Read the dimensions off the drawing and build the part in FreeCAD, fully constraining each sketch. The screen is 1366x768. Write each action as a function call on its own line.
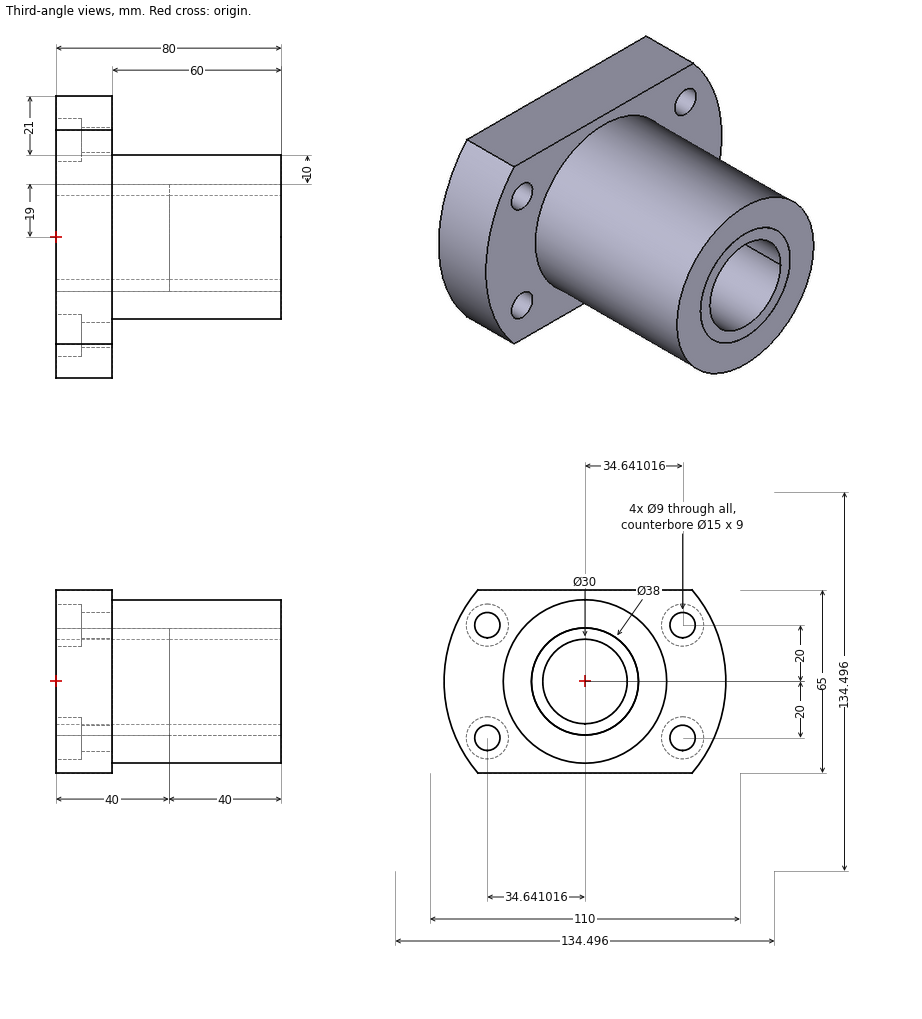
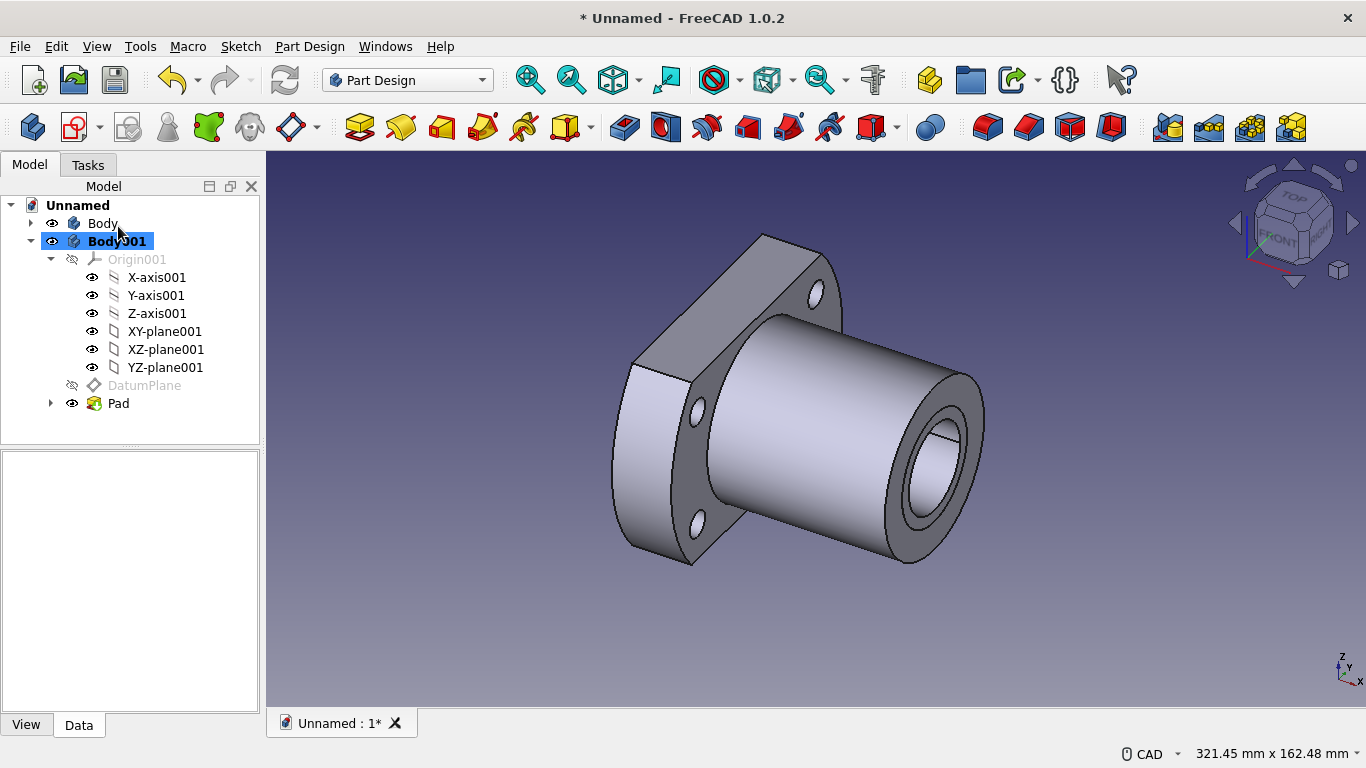
click(531, 80)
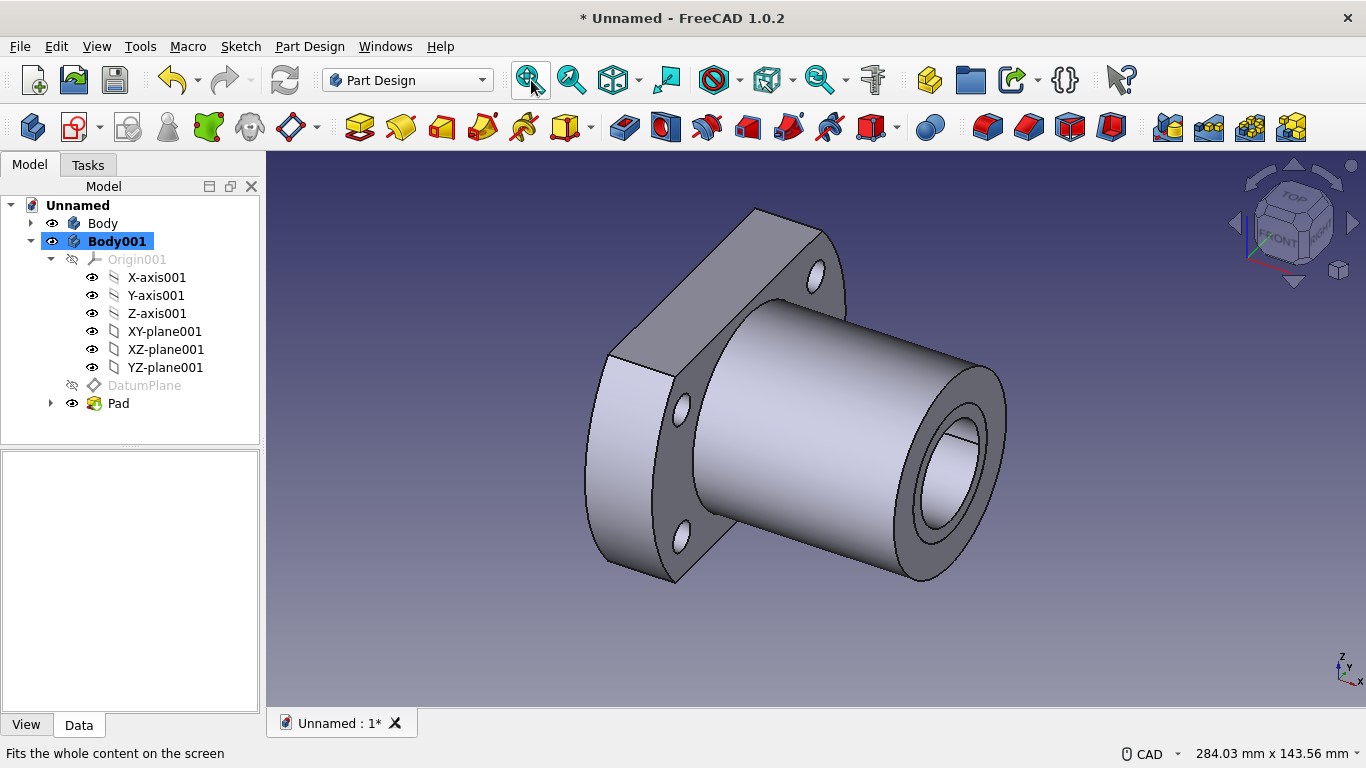
click(33, 128)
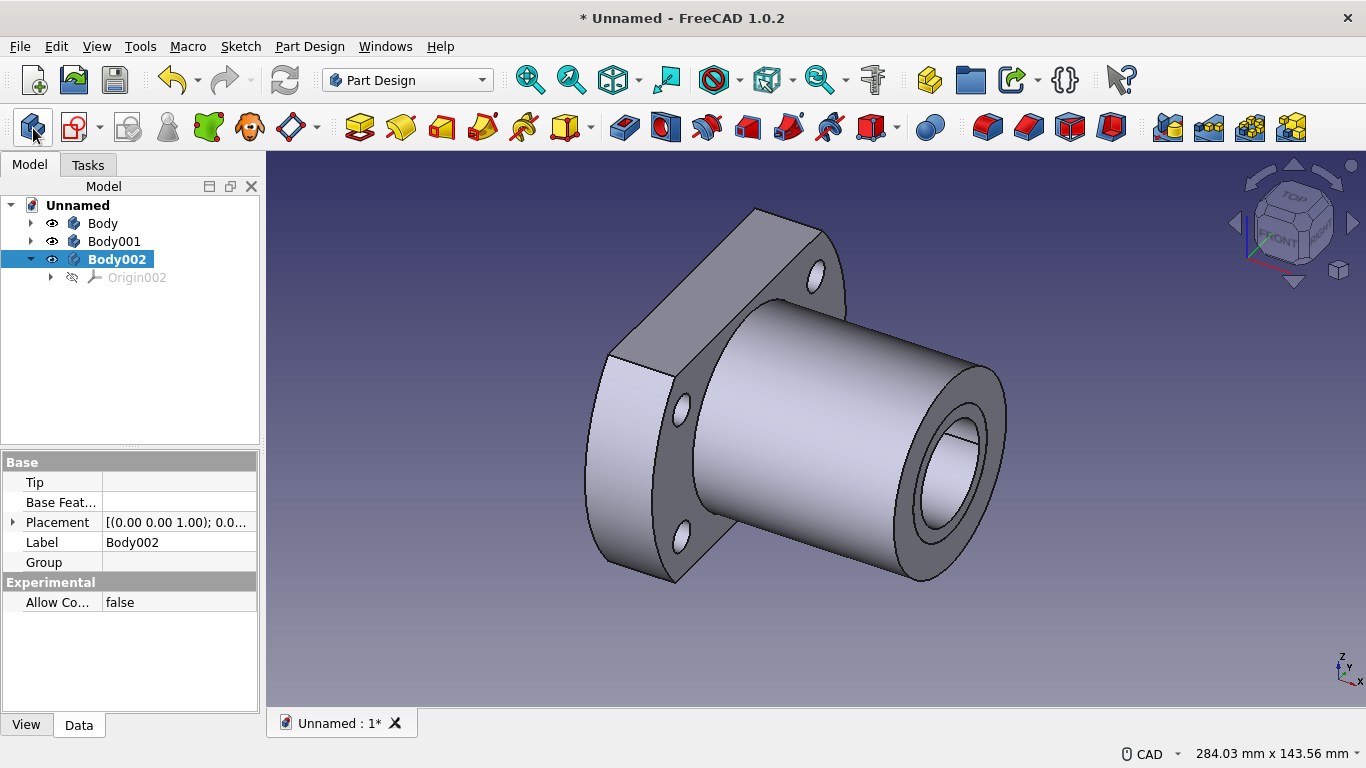
click(306, 667)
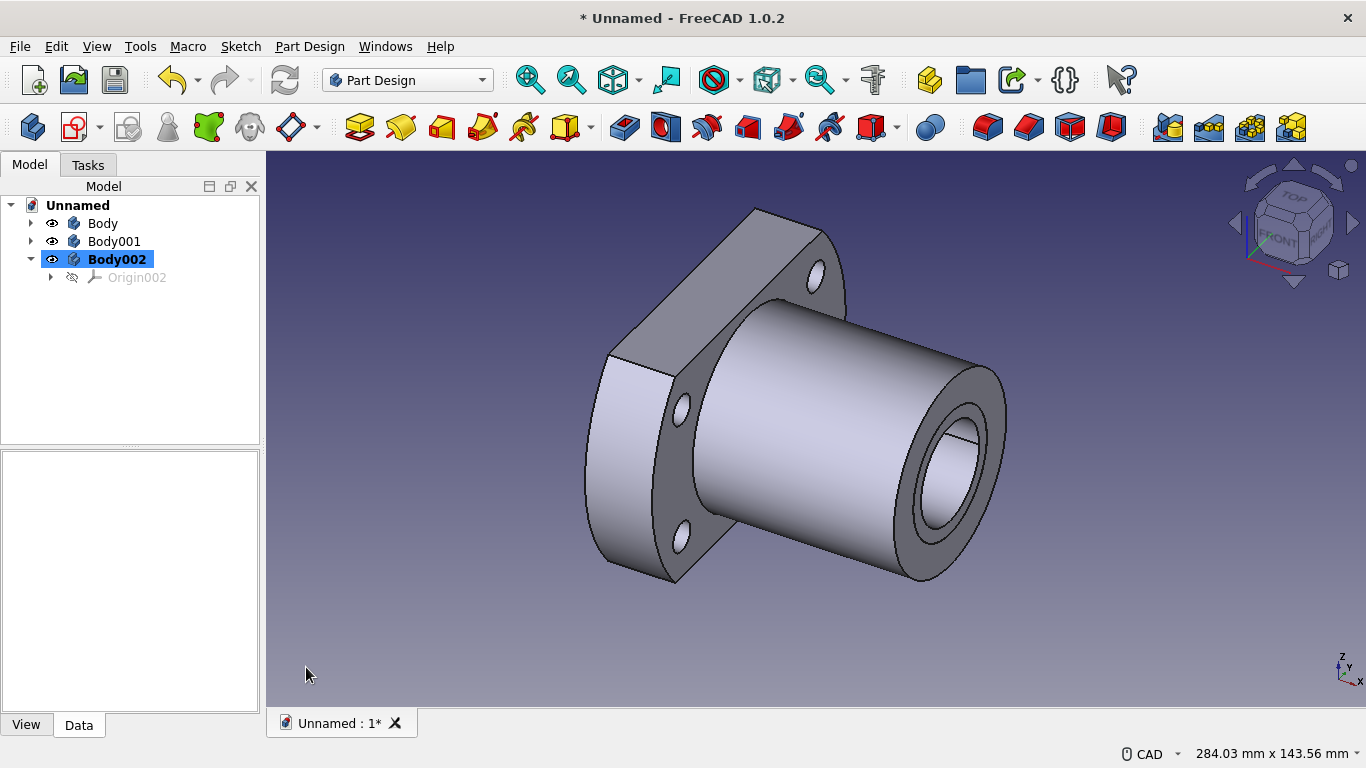
click(74, 128)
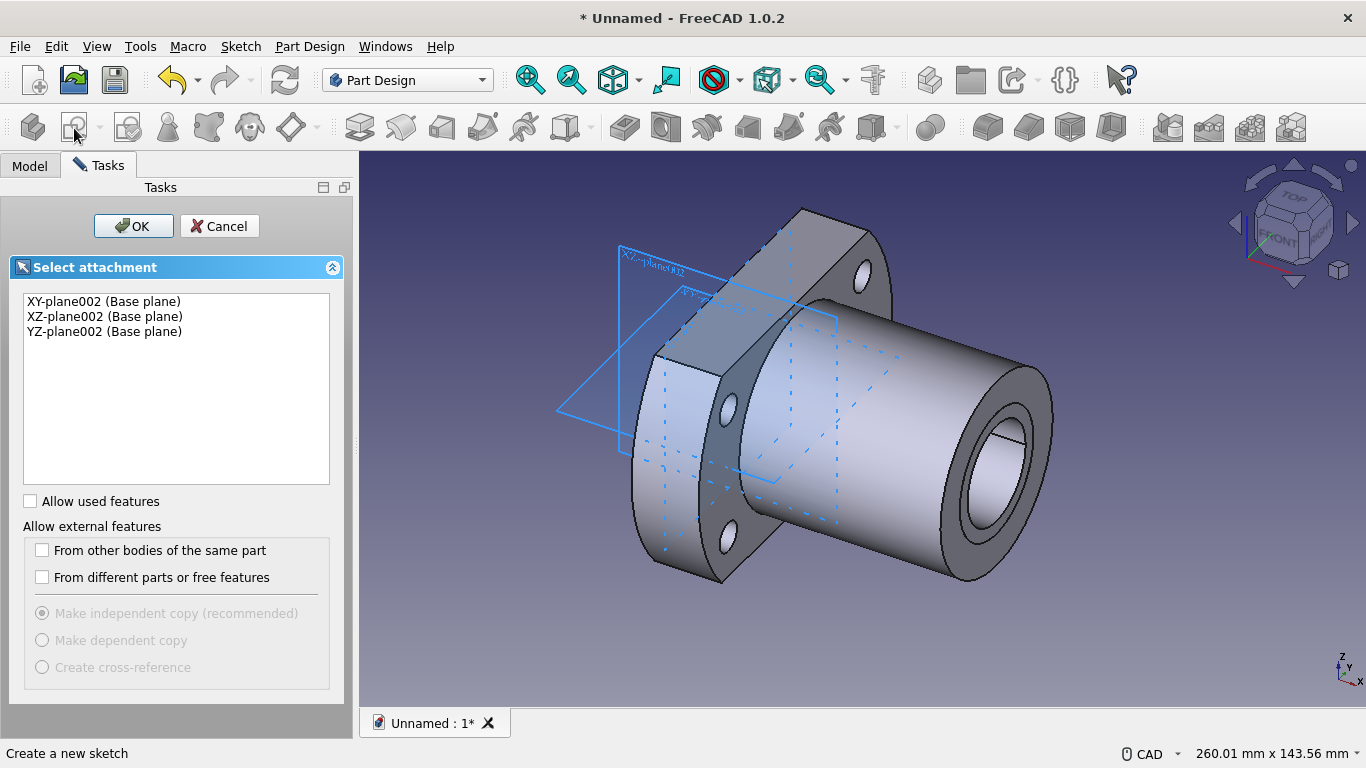
click(84, 332)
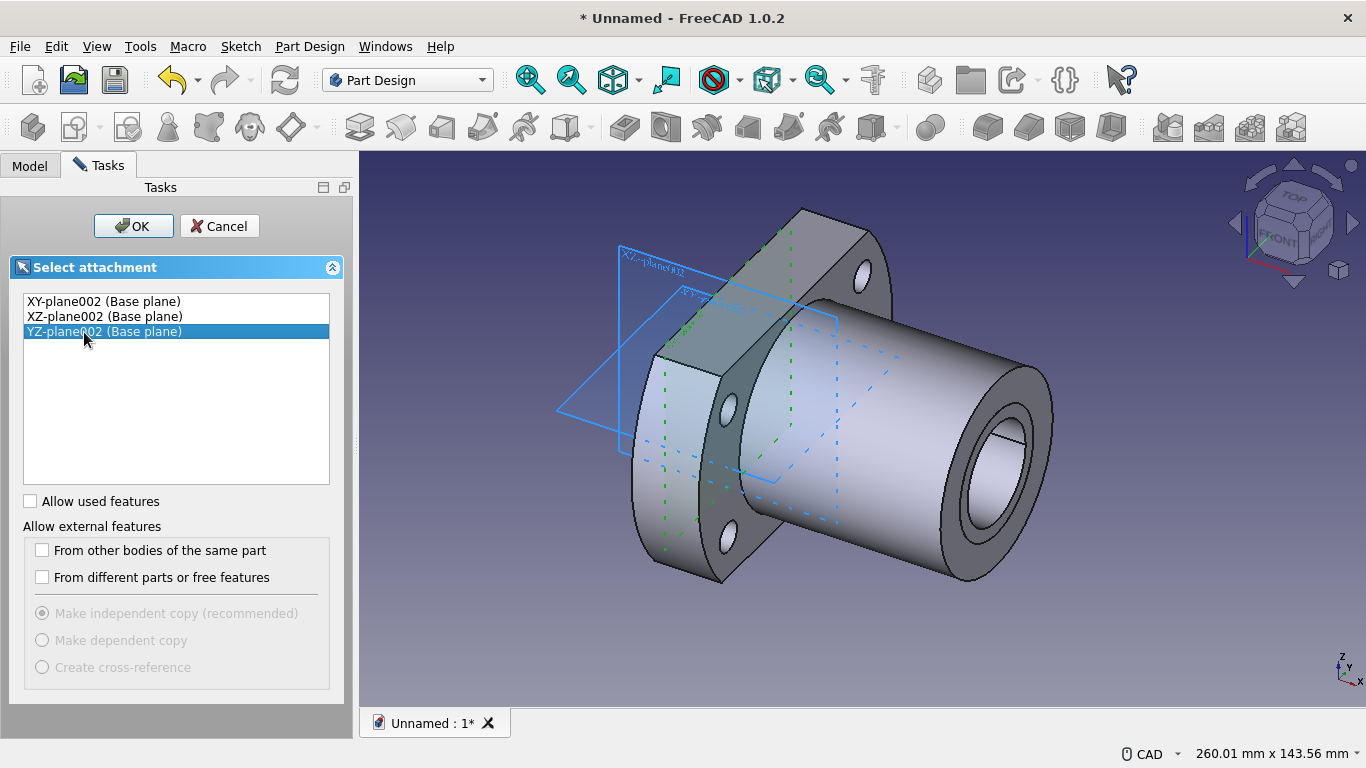
click(134, 226)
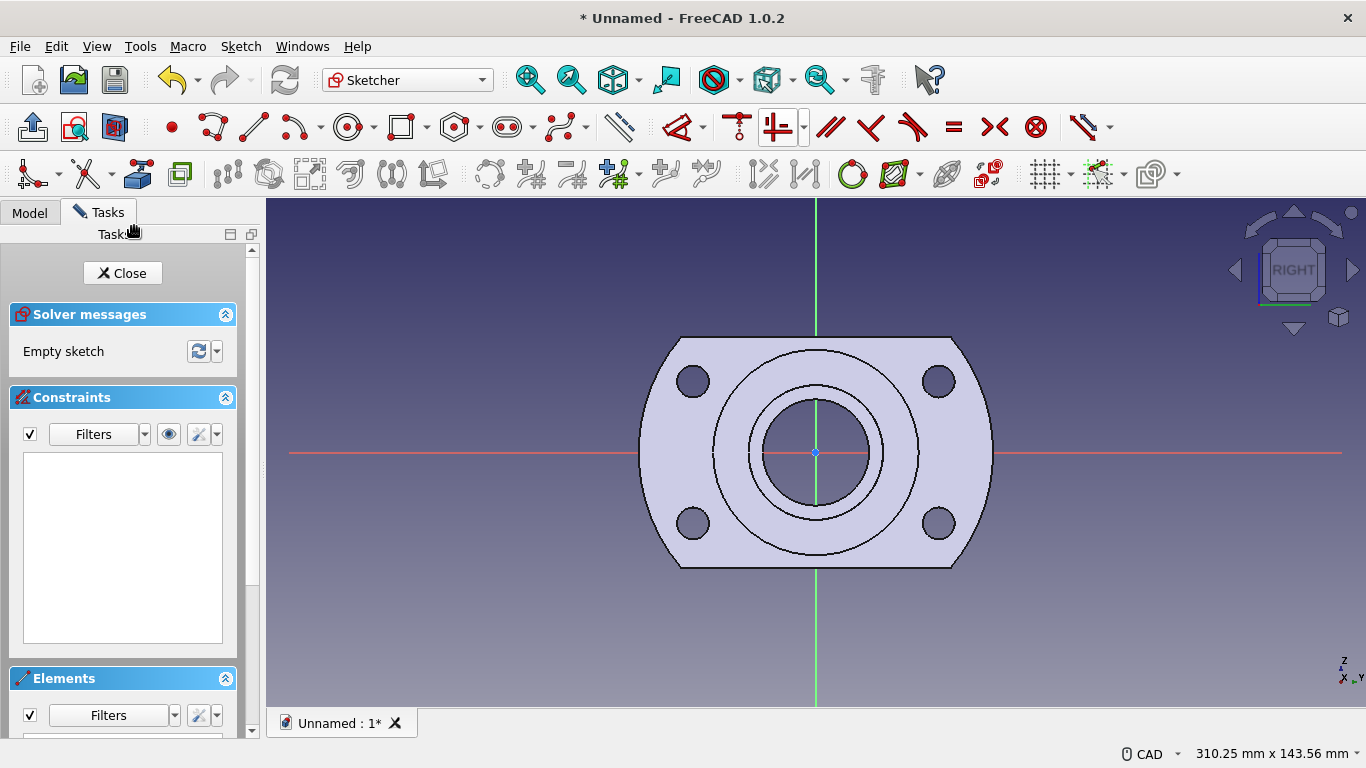
scroll(872, 452, up, 4)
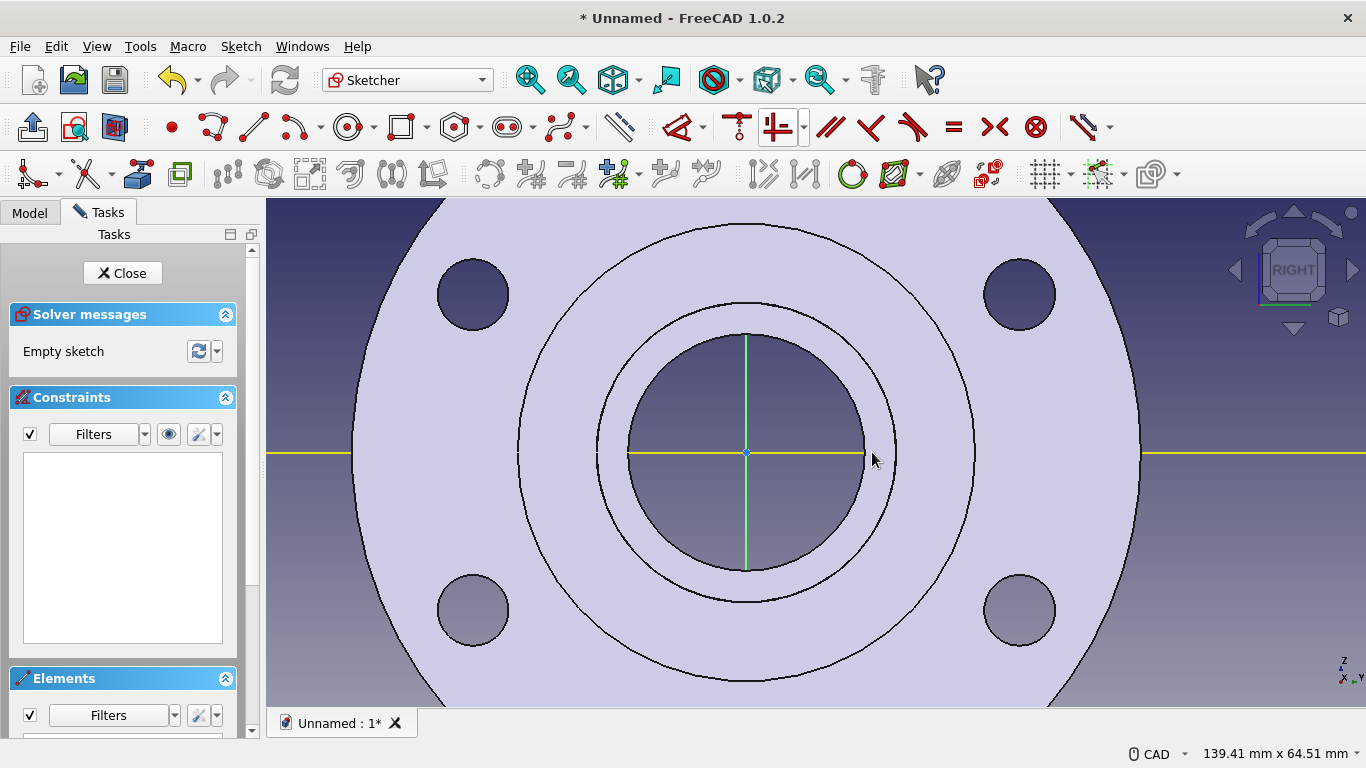
key(g)
key(c)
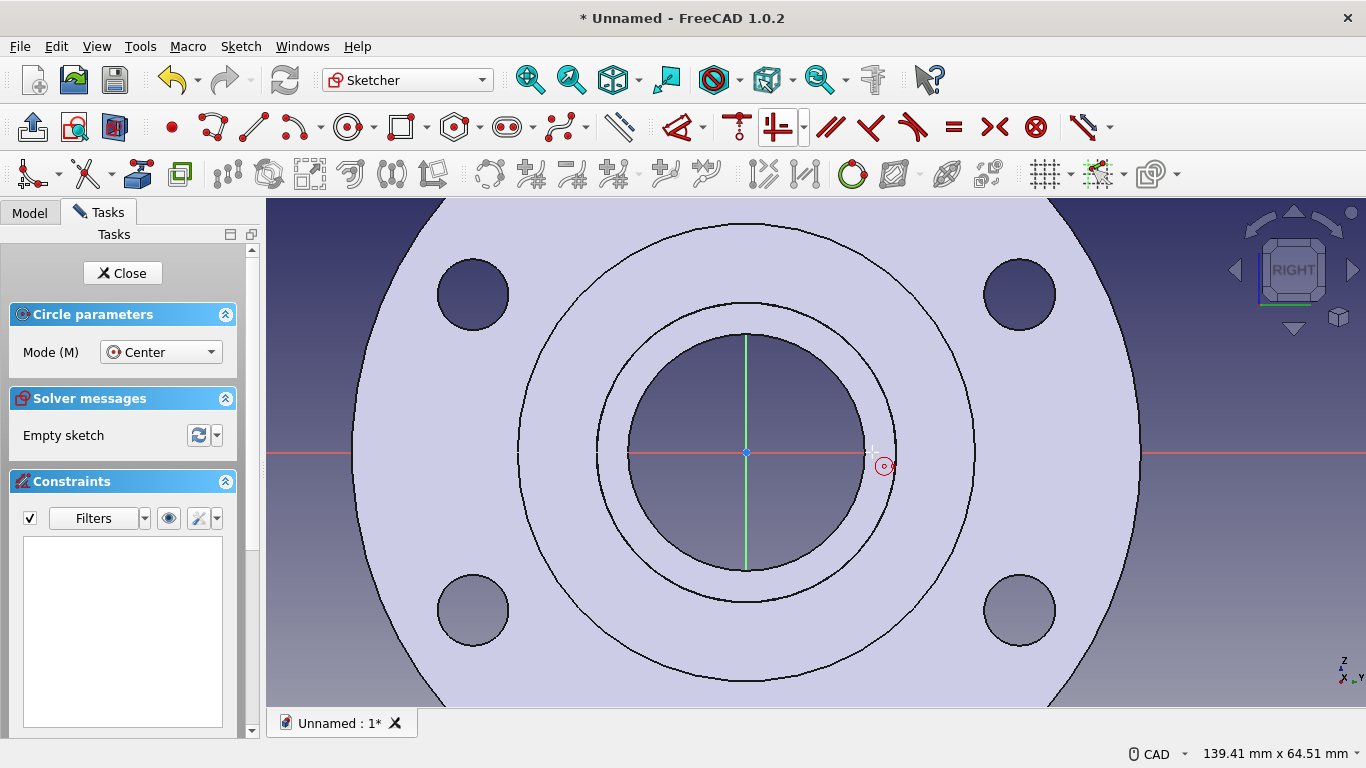
click(746, 452)
click(852, 346)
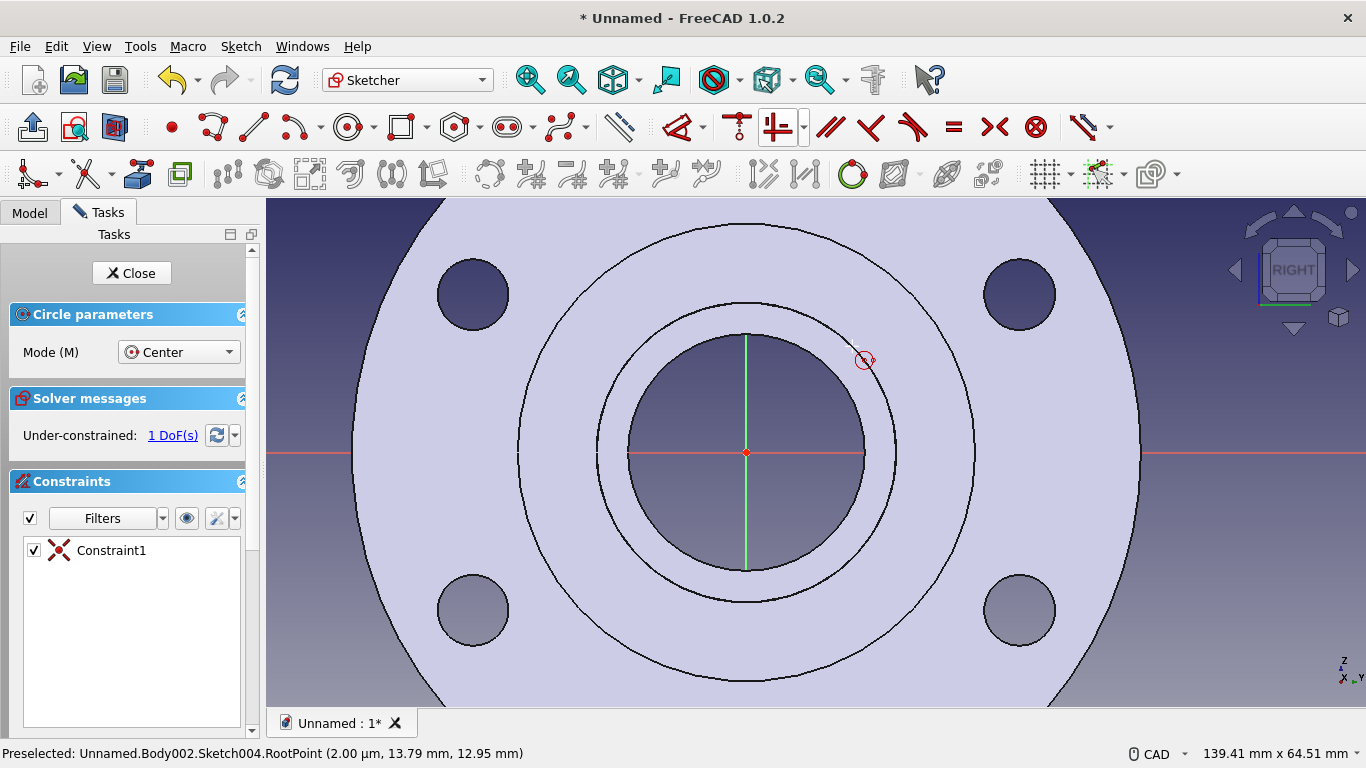
click(746, 452)
click(830, 369)
key(Escape)